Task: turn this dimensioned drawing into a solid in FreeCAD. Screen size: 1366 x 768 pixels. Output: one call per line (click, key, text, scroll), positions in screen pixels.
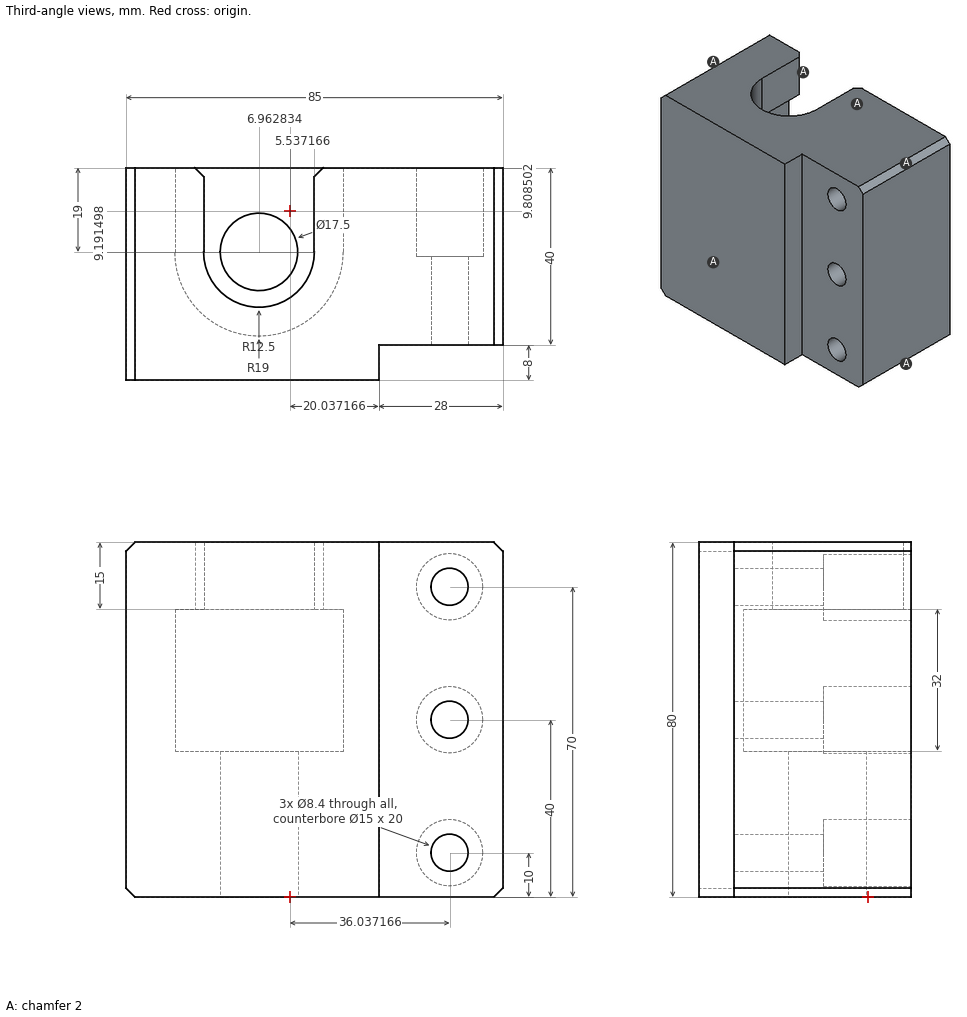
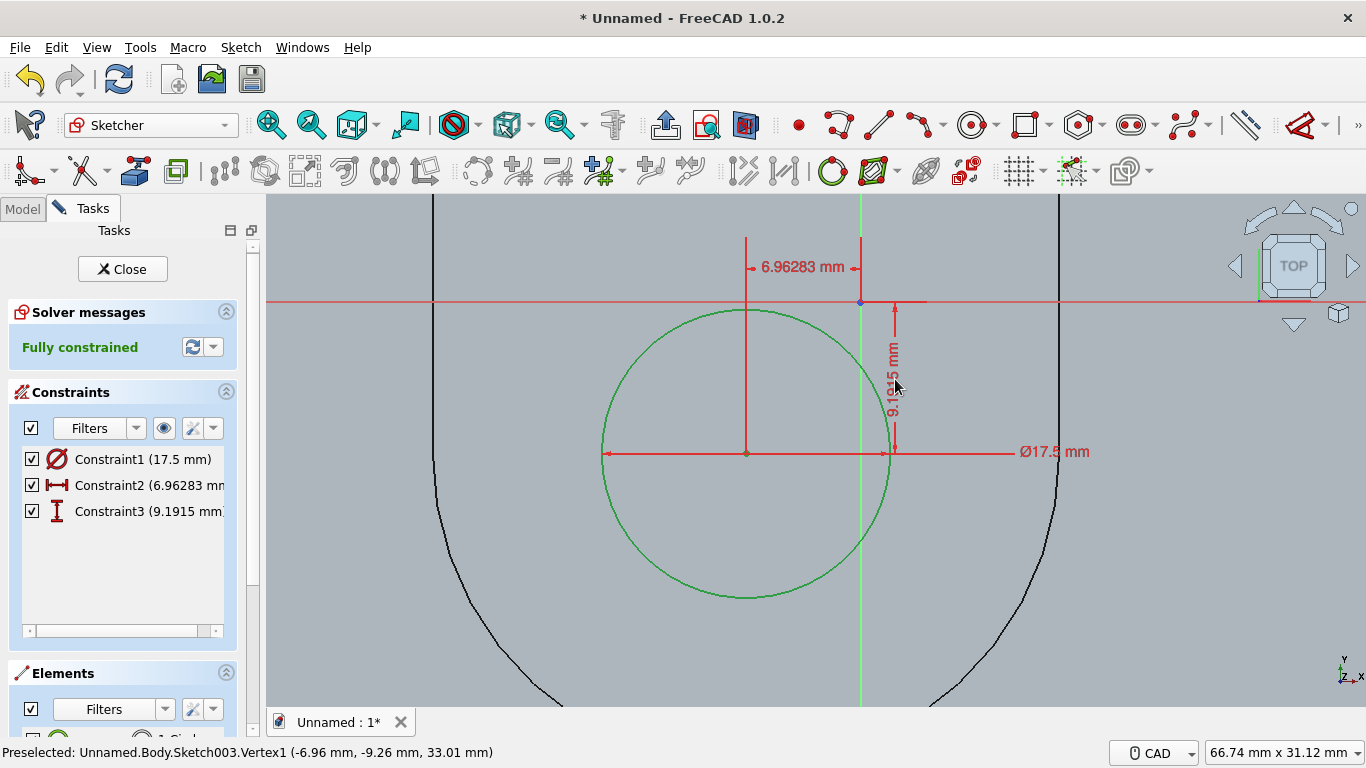
click(123, 269)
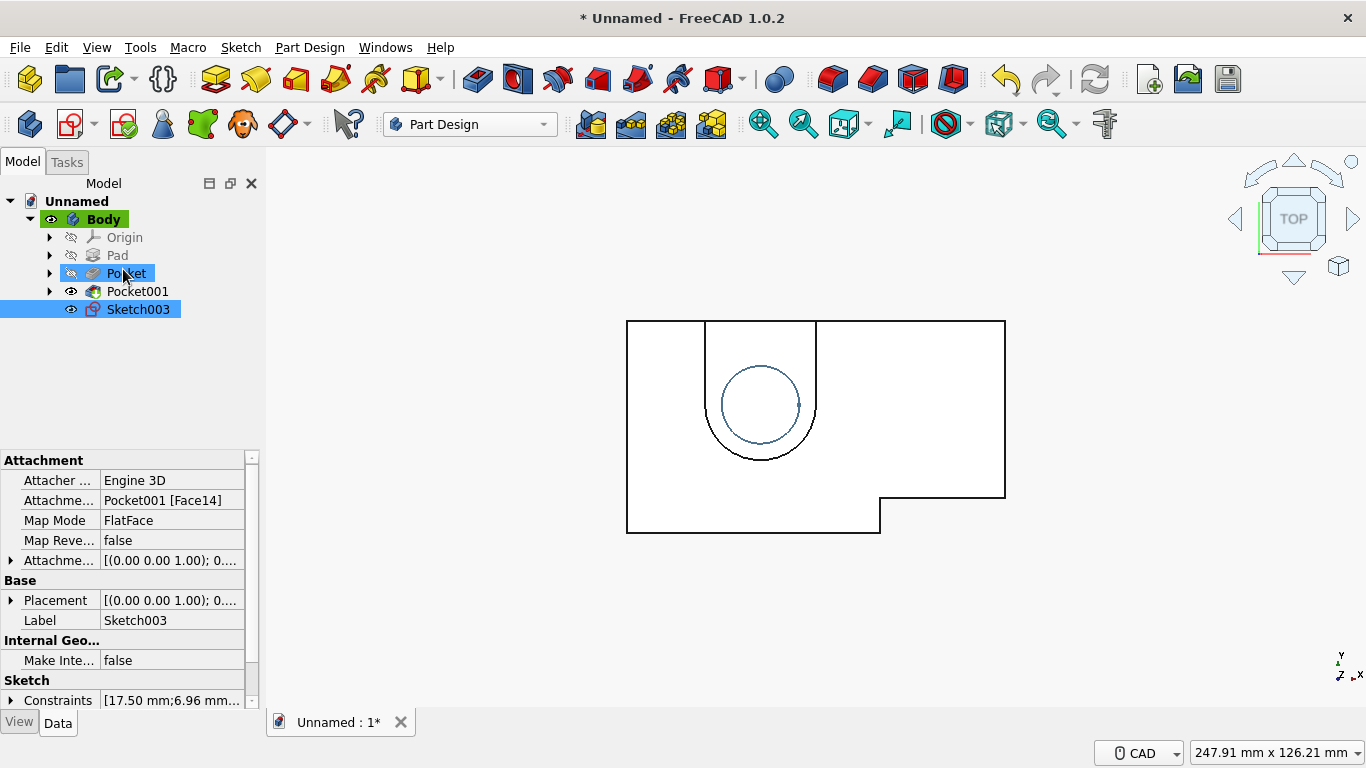
click(478, 80)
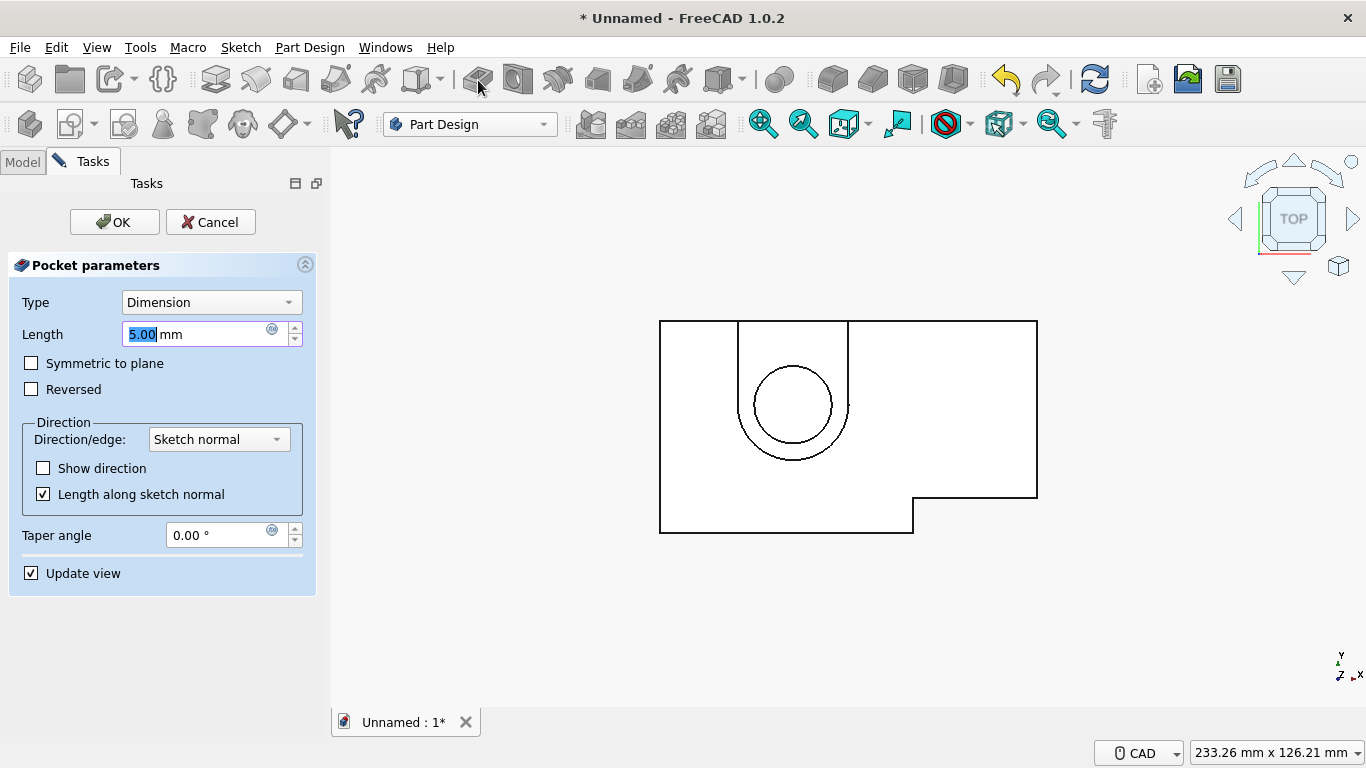
click(212, 302)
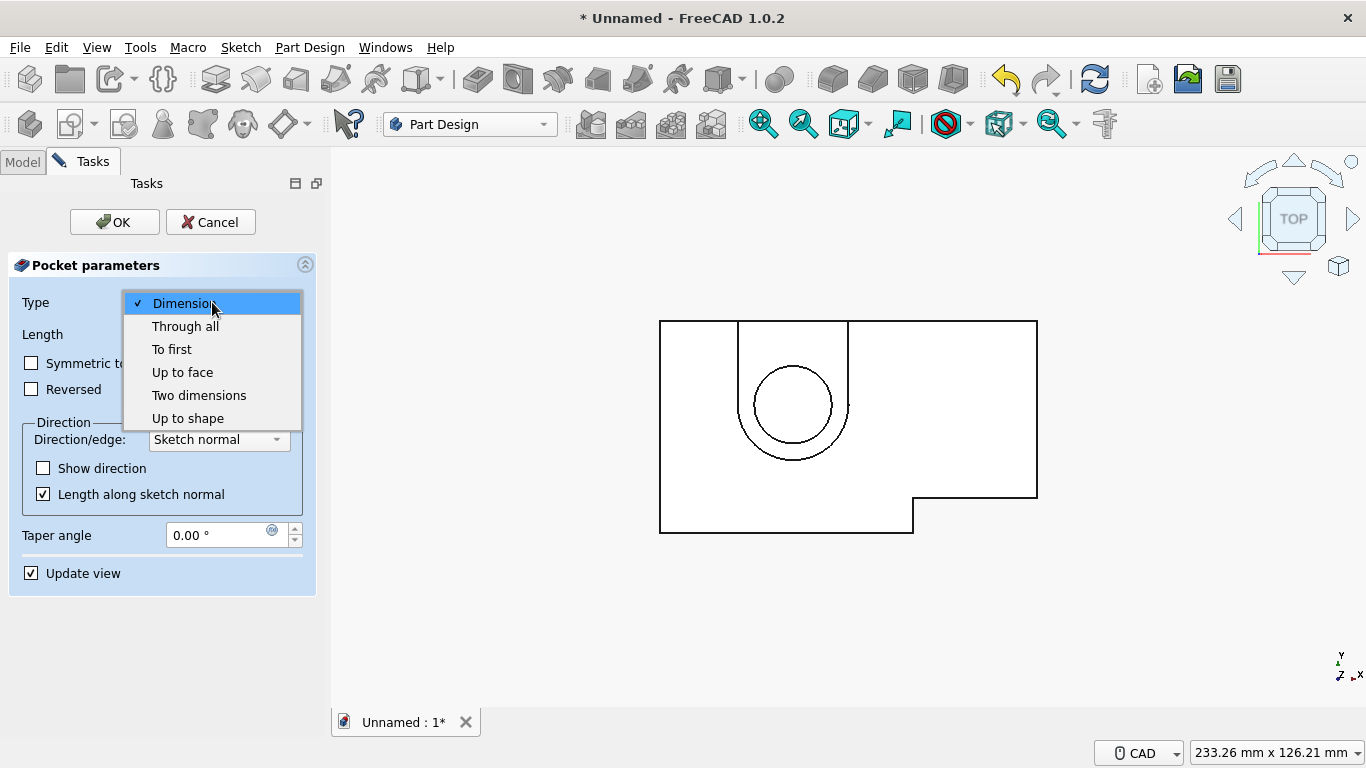
click(212, 326)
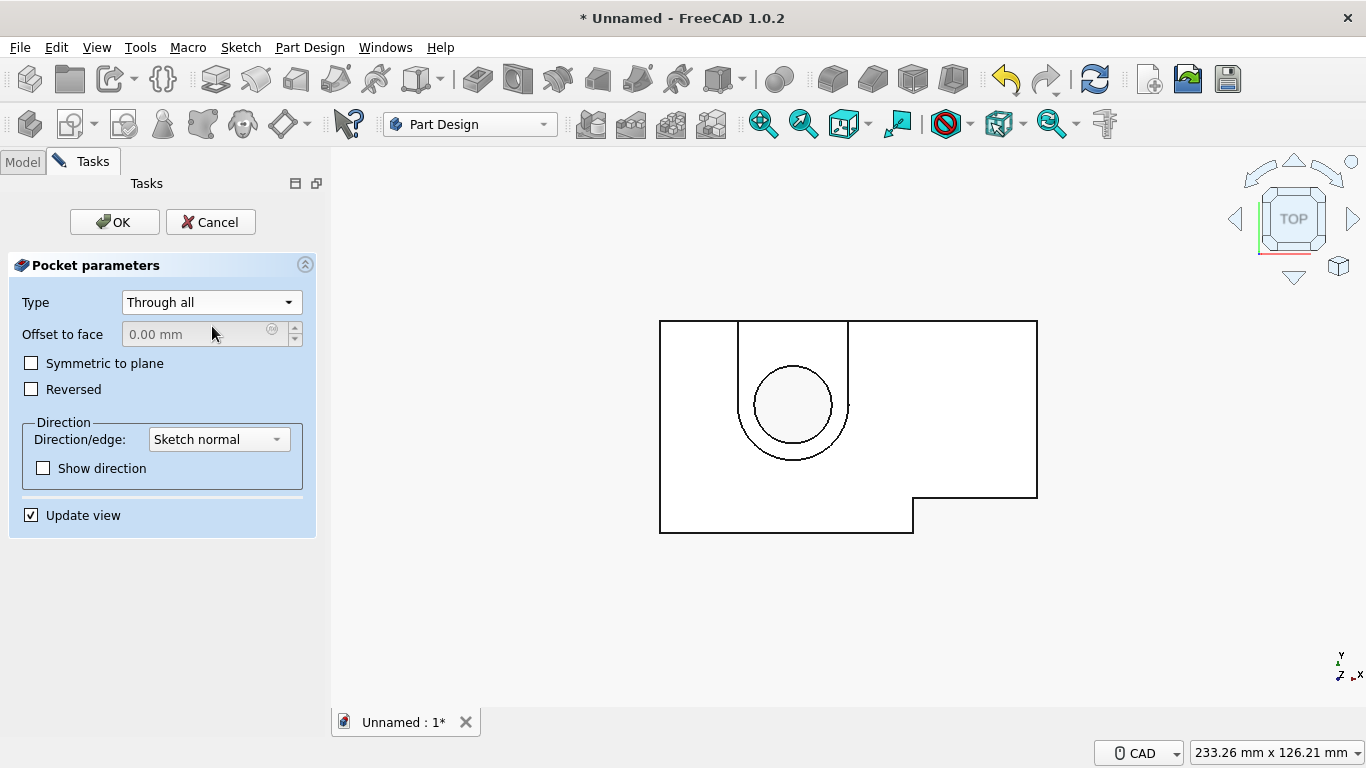
click(115, 222)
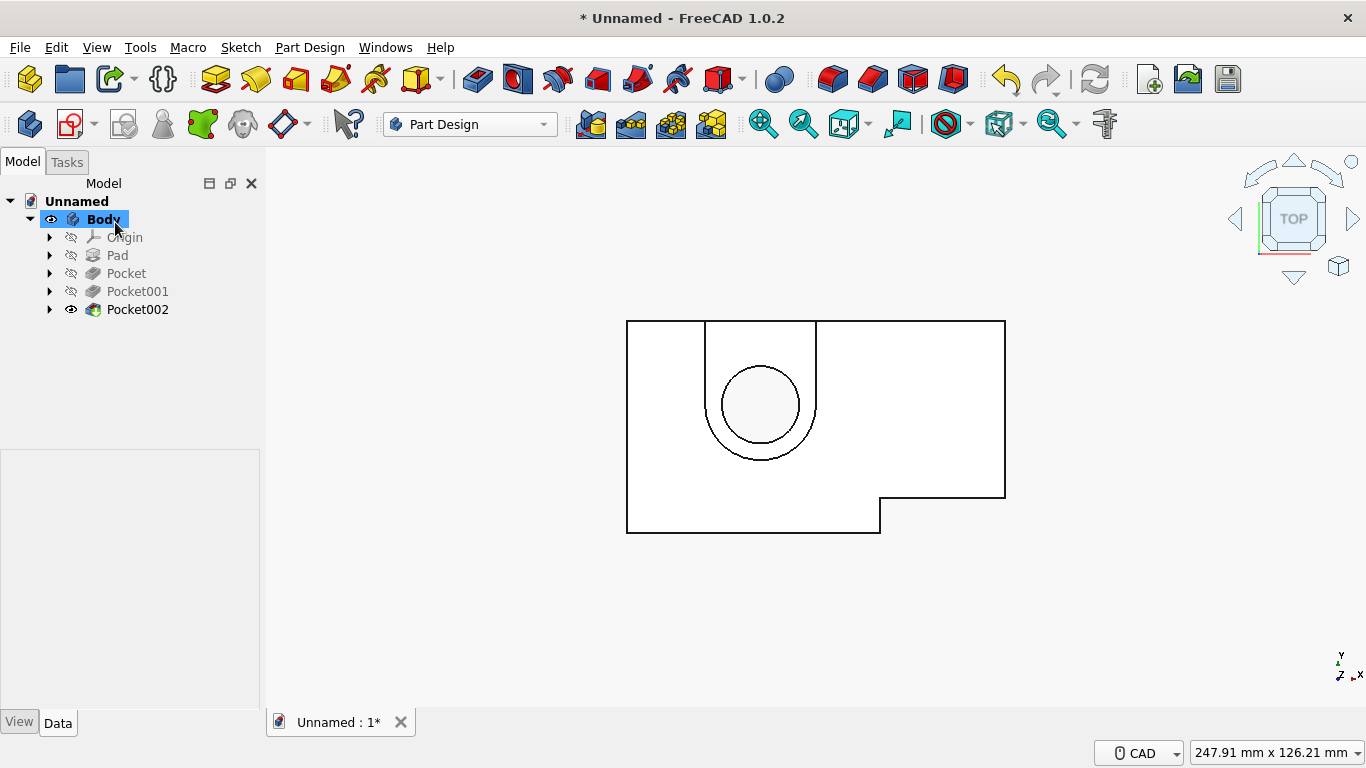
key(v)
key(f)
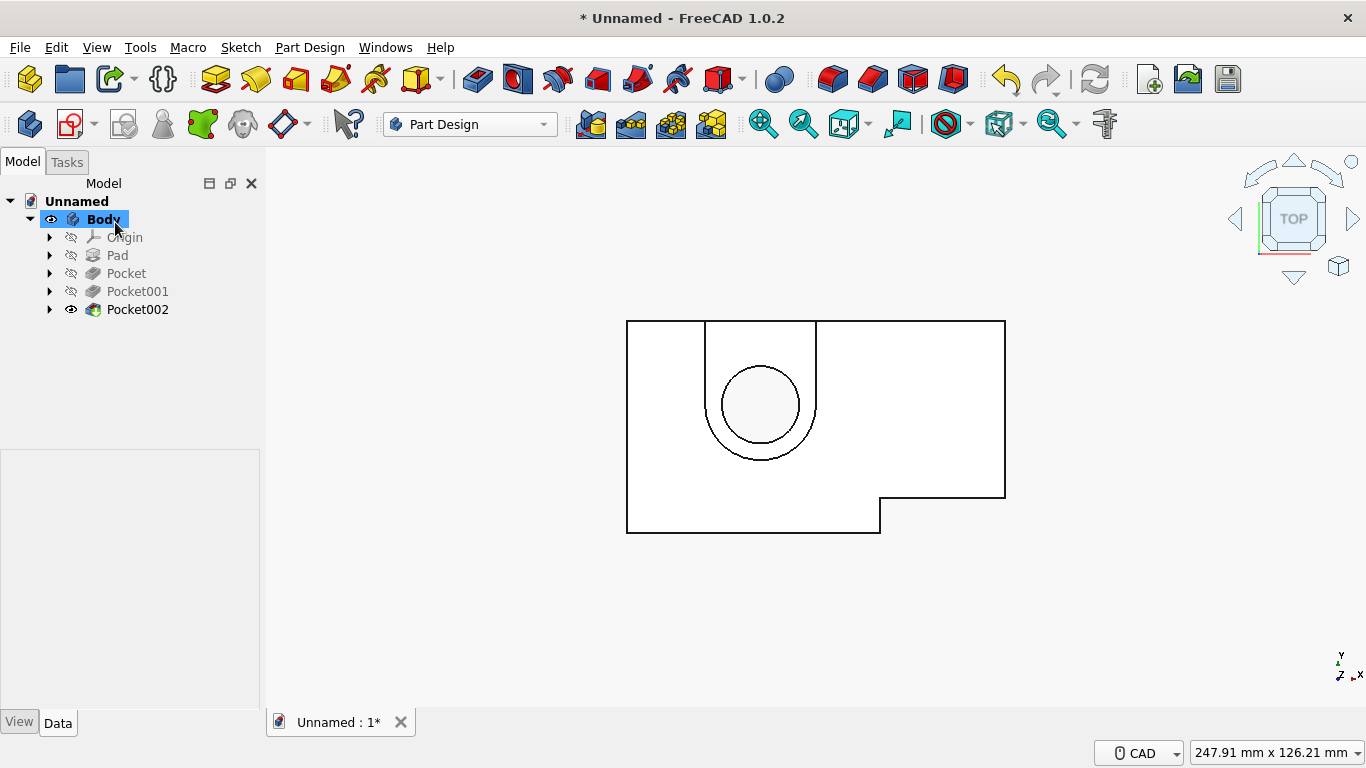
key(4)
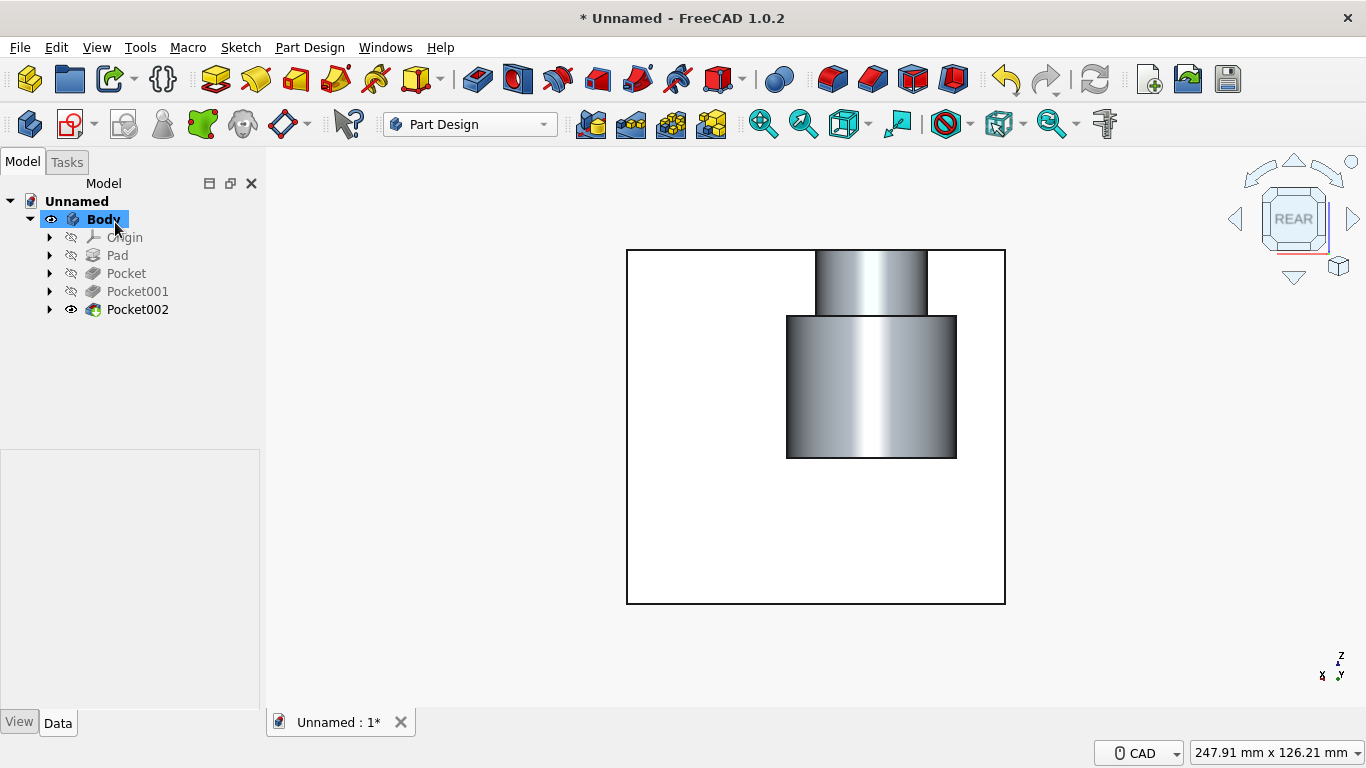
click(708, 477)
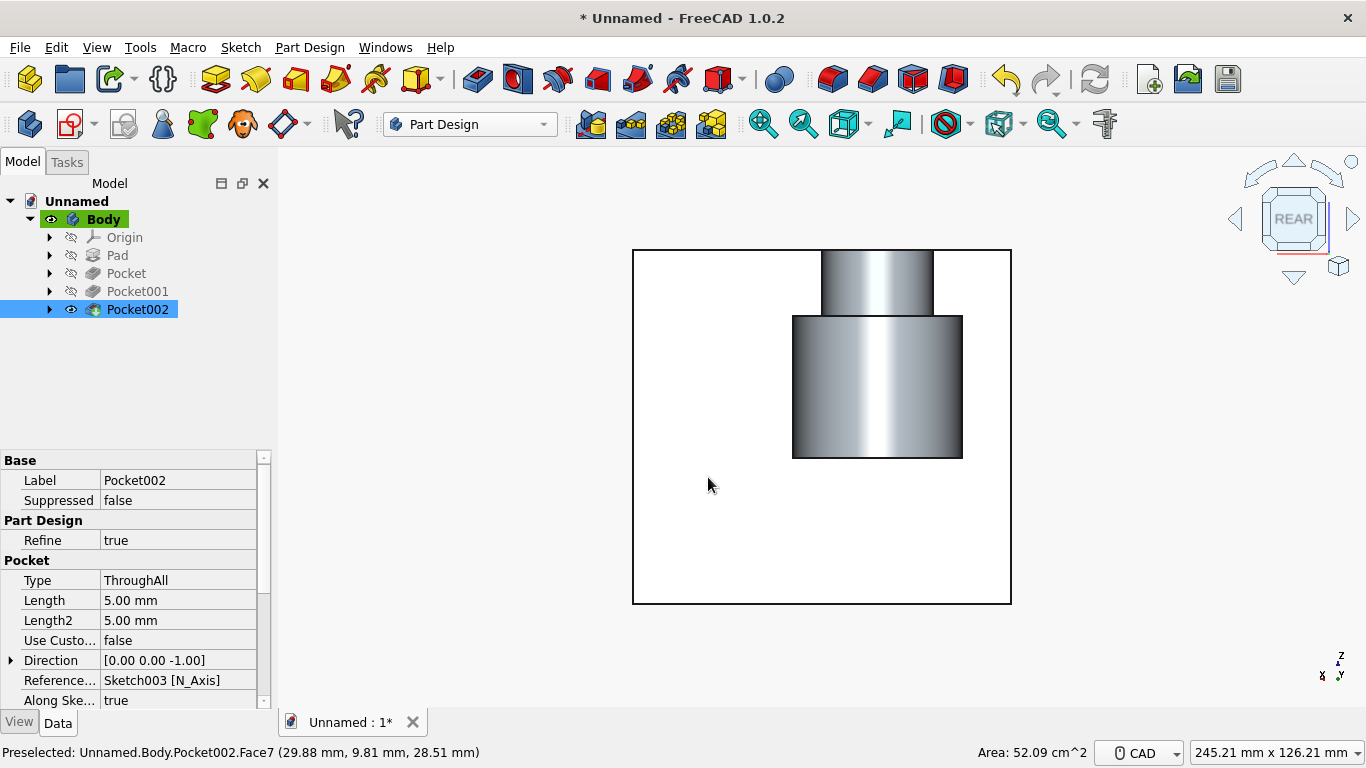
click(70, 124)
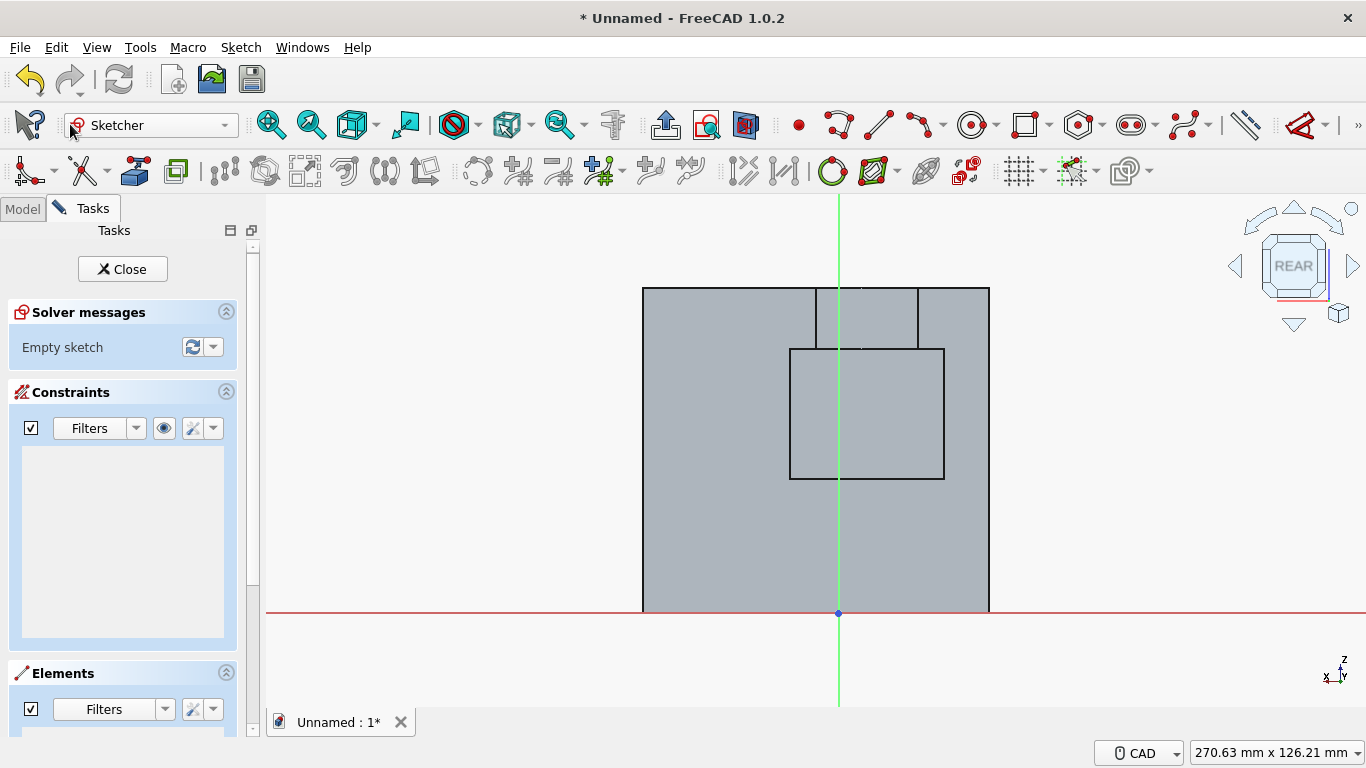
key(g)
key(c)